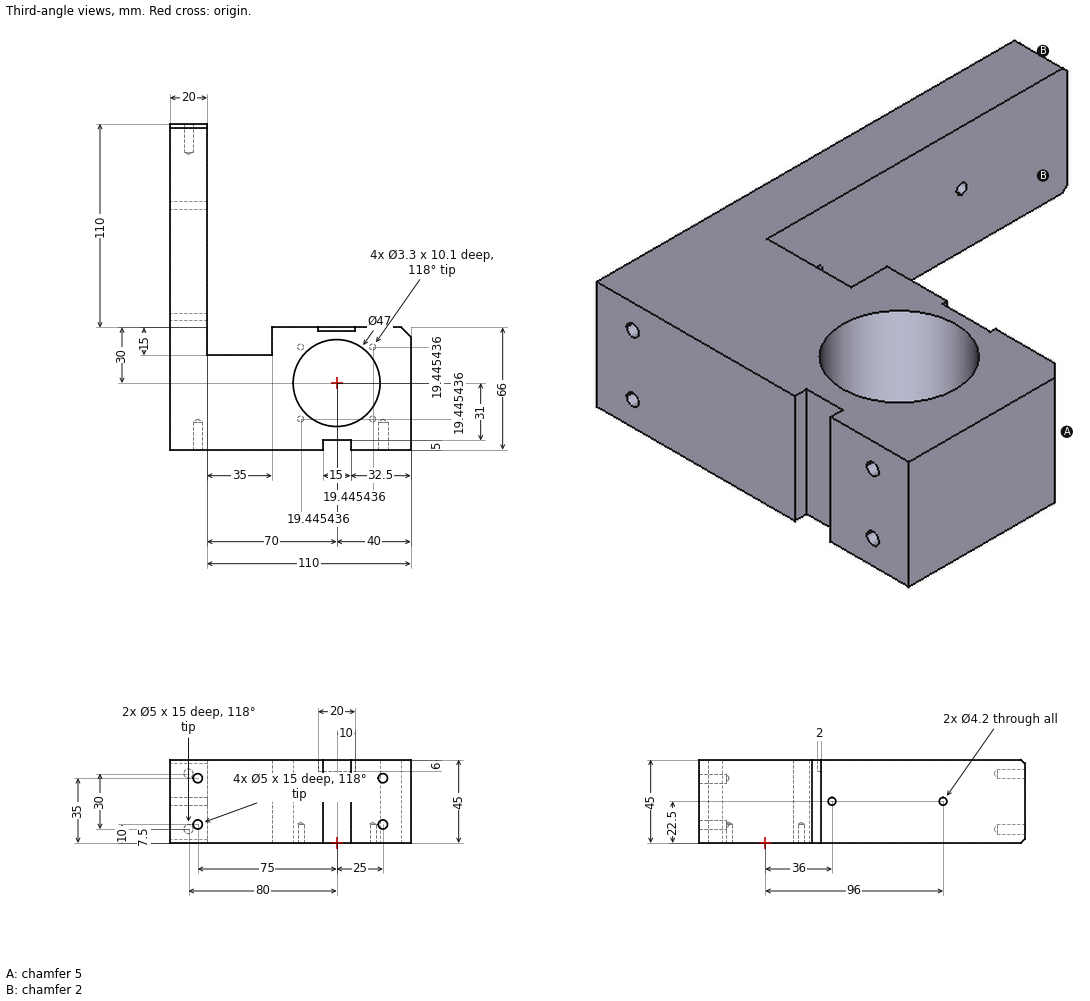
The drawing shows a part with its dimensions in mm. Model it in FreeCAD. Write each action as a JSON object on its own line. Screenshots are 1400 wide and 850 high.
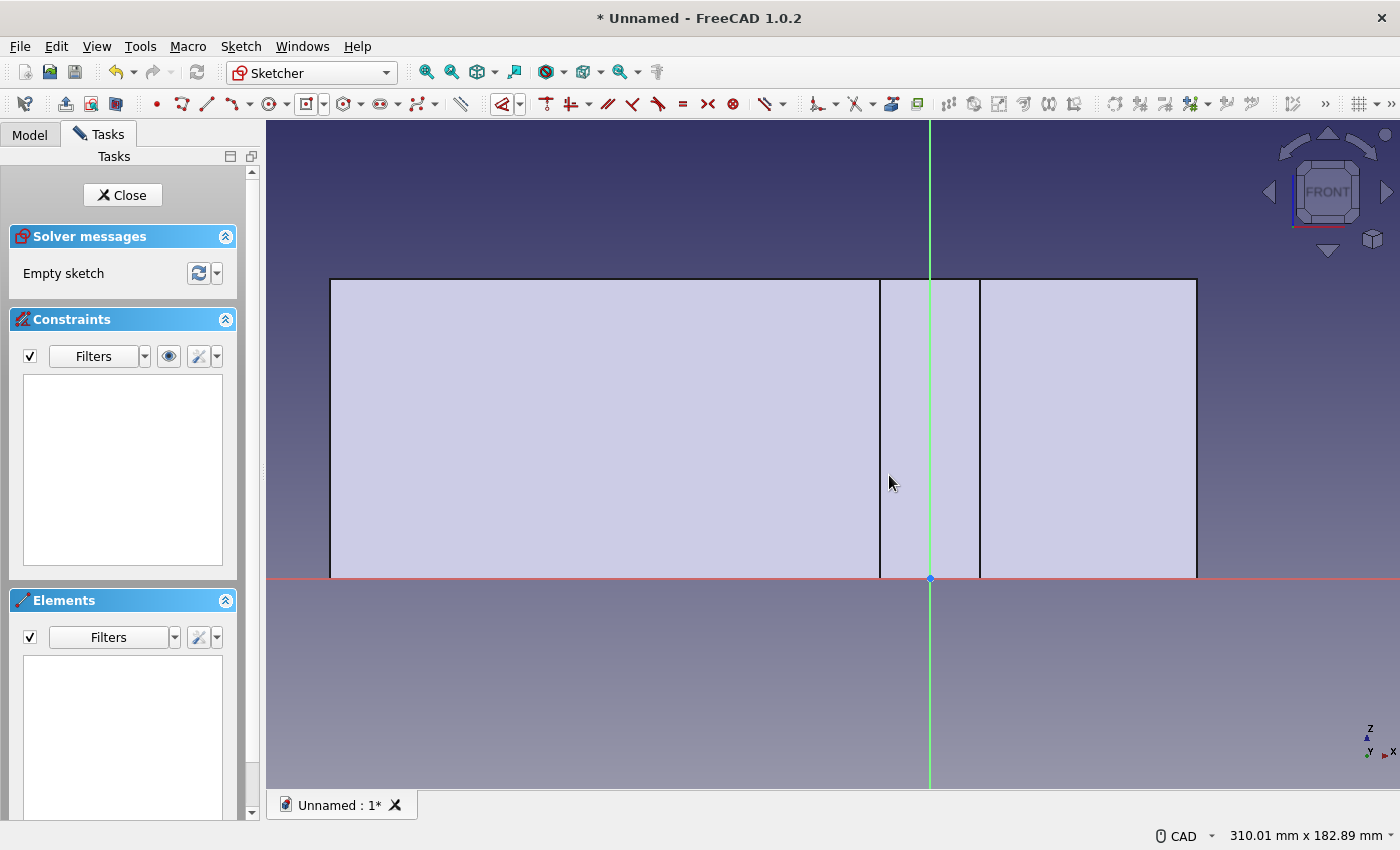
{"action": "left_click", "coordinate": [268, 104]}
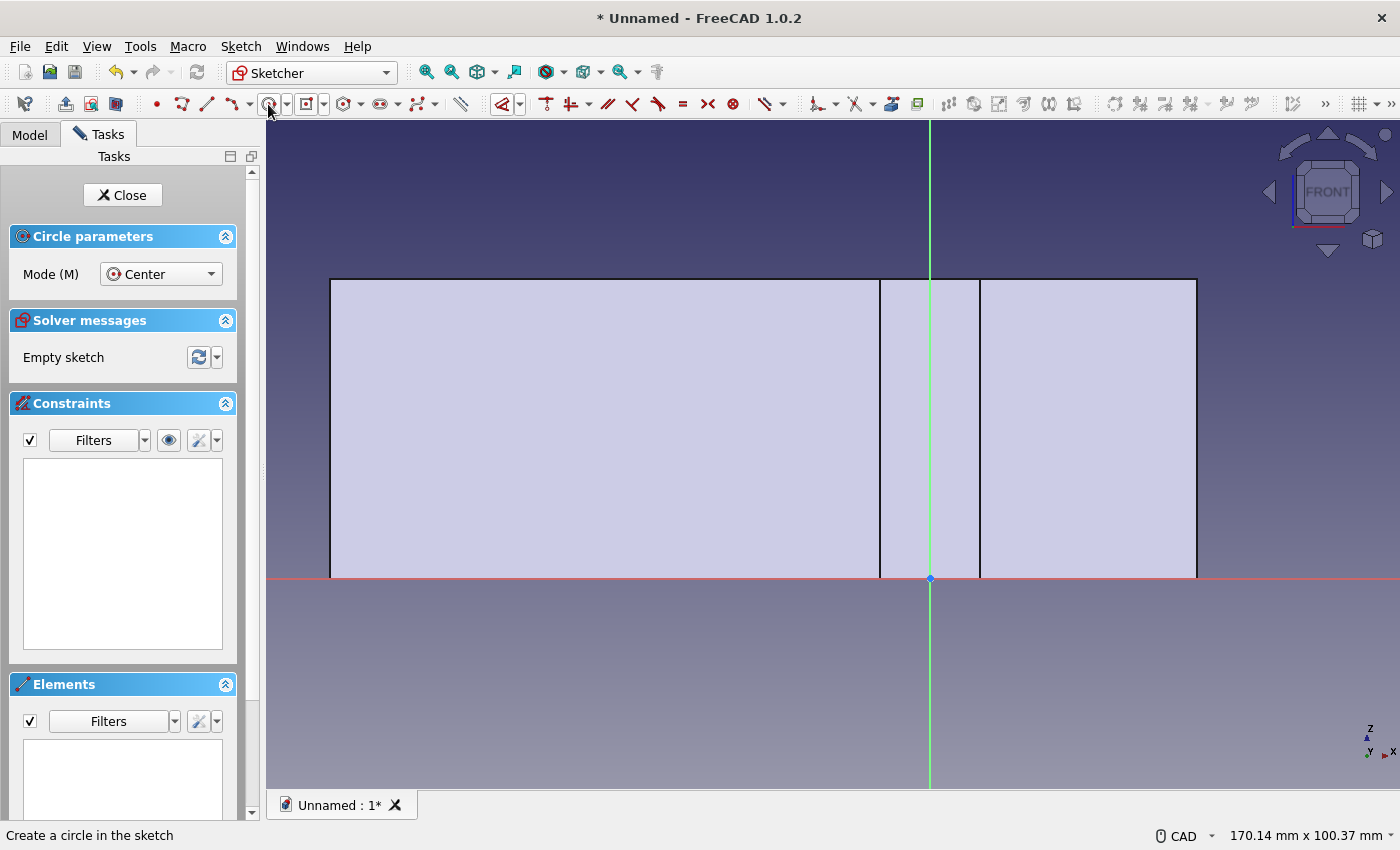
{"action": "scroll", "coordinate": [430, 512], "scroll_direction": "up", "scroll_amount": 2}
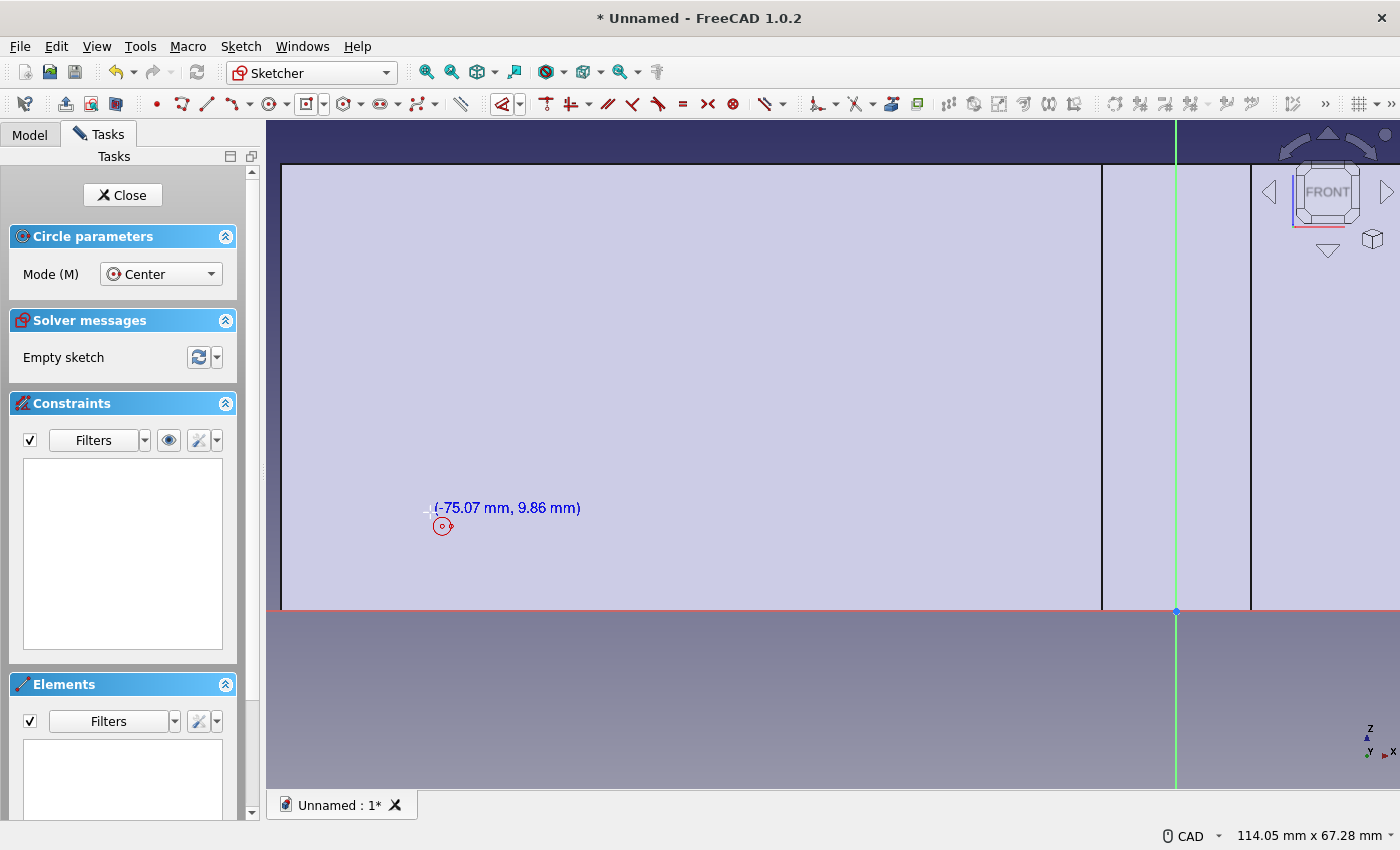
{"action": "left_click", "coordinate": [431, 512]}
{"action": "left_click", "coordinate": [448, 494]}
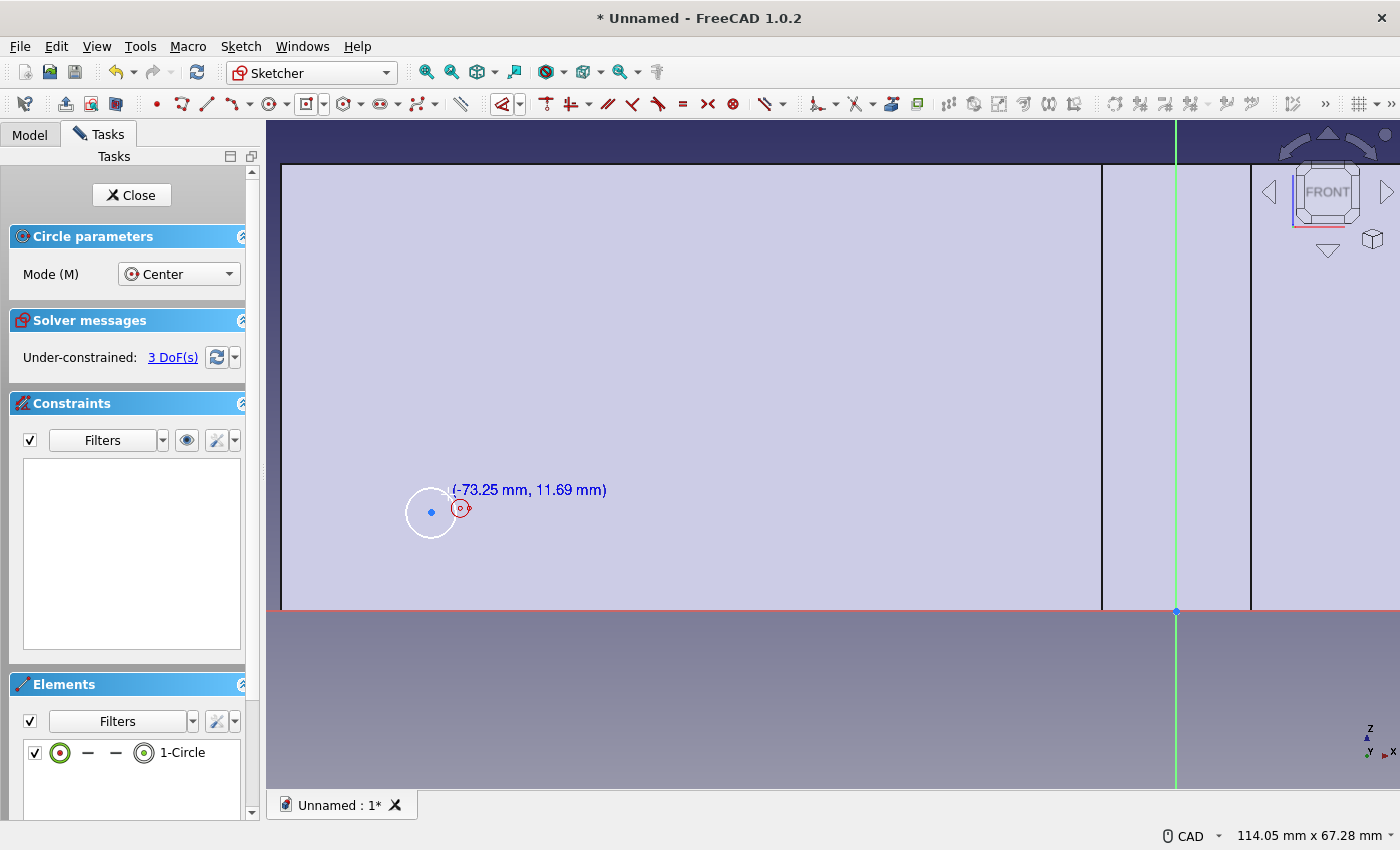
{"action": "scroll", "coordinate": [433, 515], "scroll_direction": "down", "scroll_amount": 2}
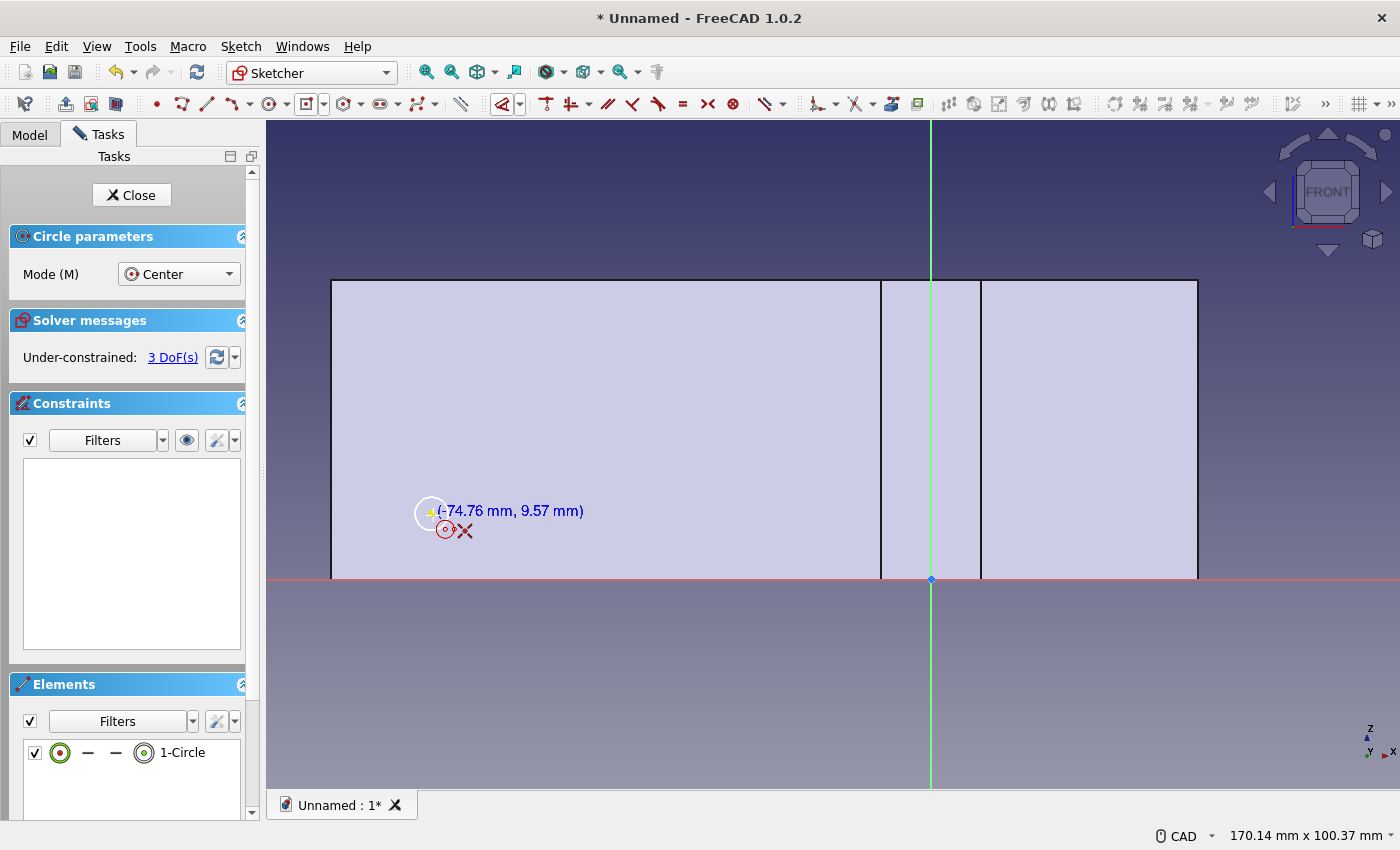
{"action": "scroll", "coordinate": [1098, 513], "scroll_direction": "up", "scroll_amount": 2}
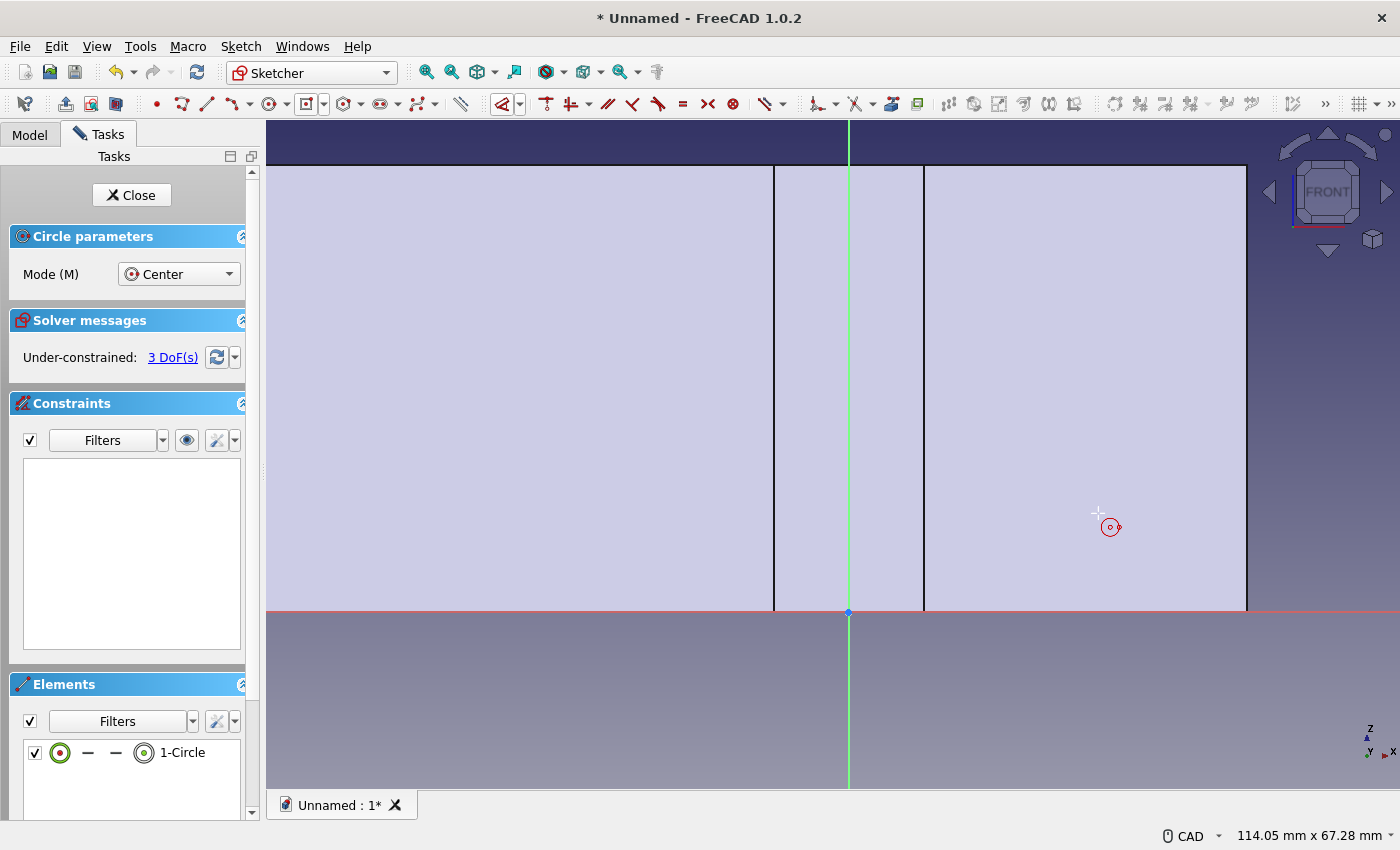
{"action": "left_click", "coordinate": [1098, 513]}
{"action": "left_click", "coordinate": [1115, 495]}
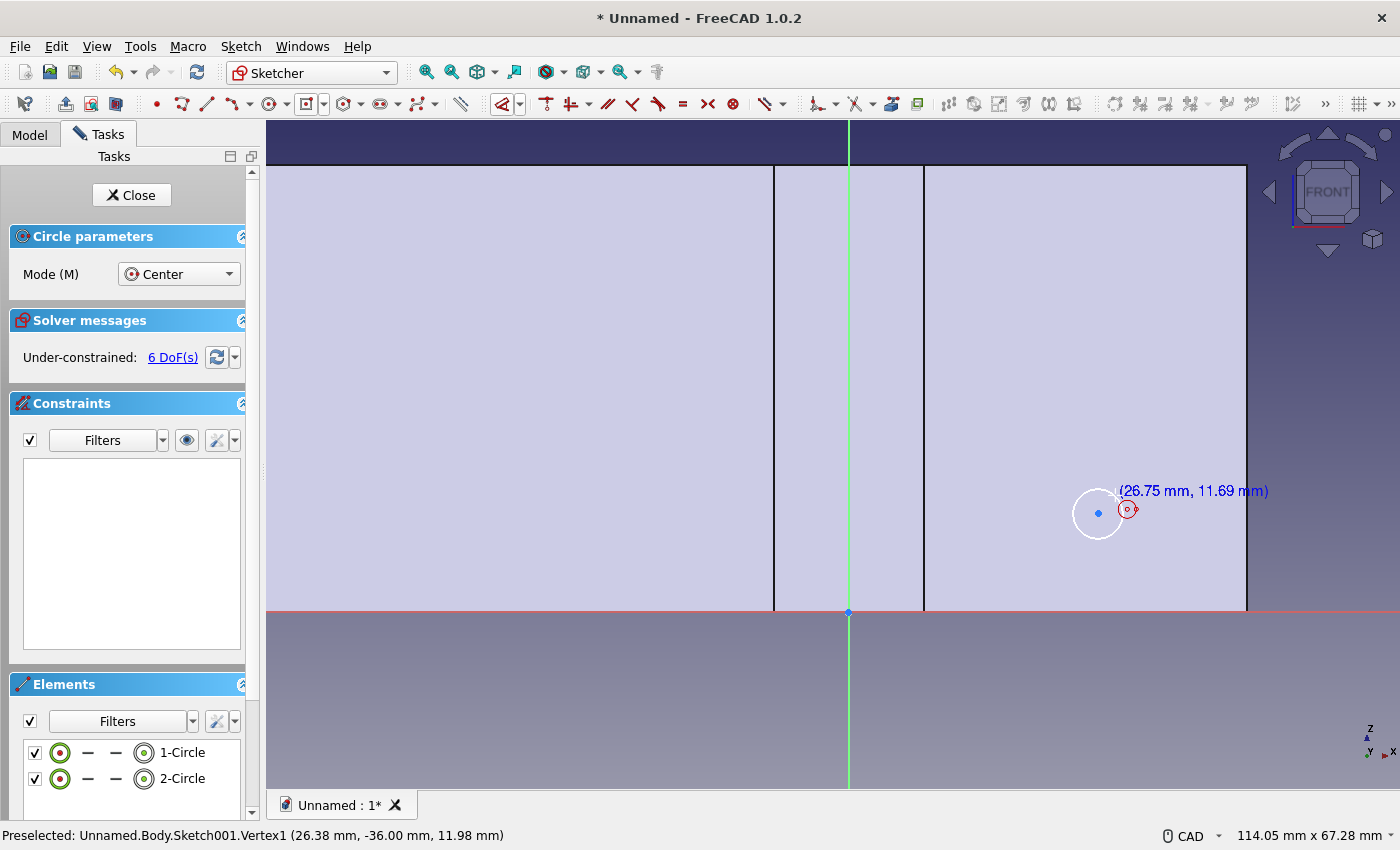
{"action": "scroll", "coordinate": [1098, 513], "scroll_direction": "down", "scroll_amount": 2}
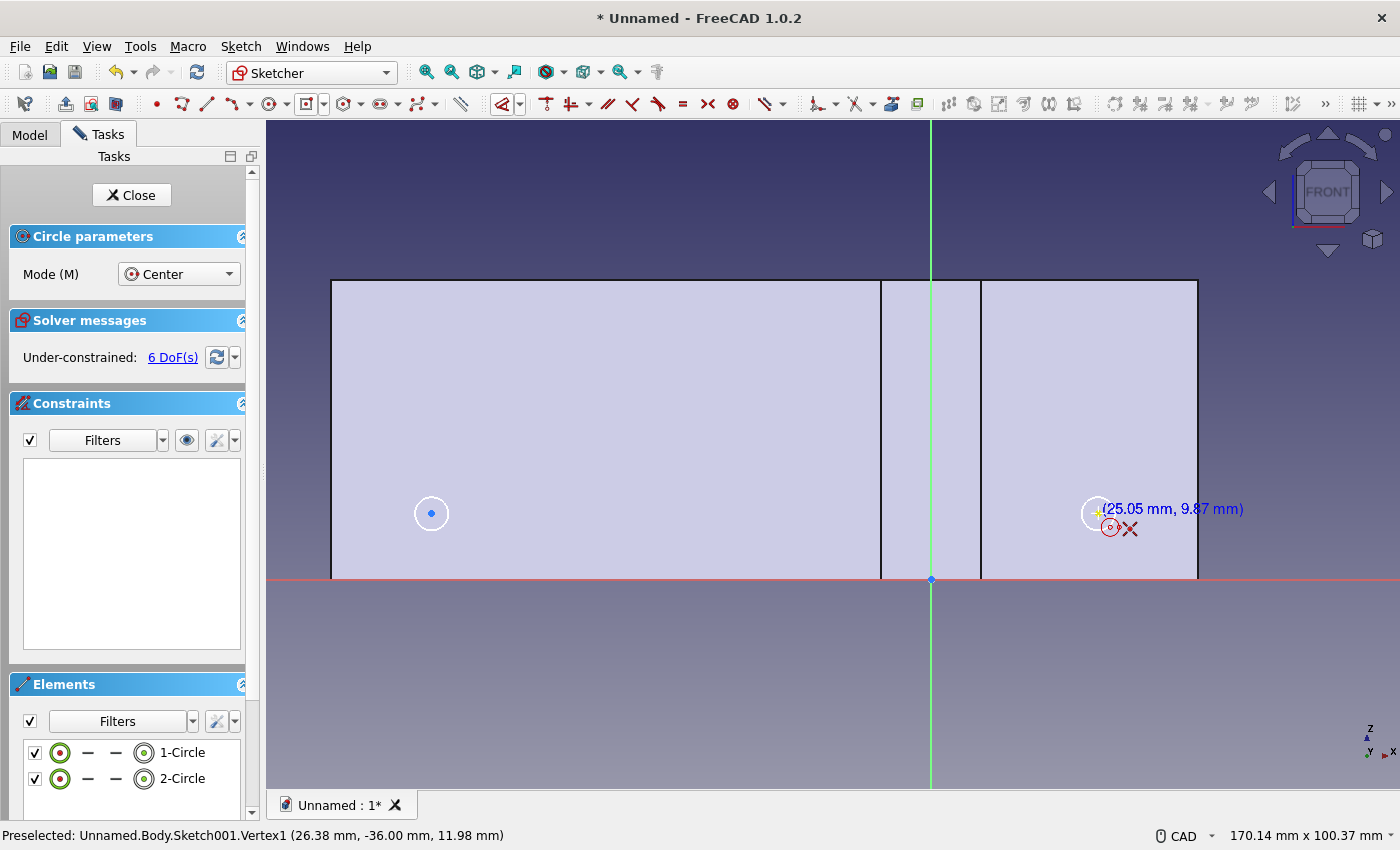
{"action": "scroll", "coordinate": [431, 346], "scroll_direction": "up", "scroll_amount": 2}